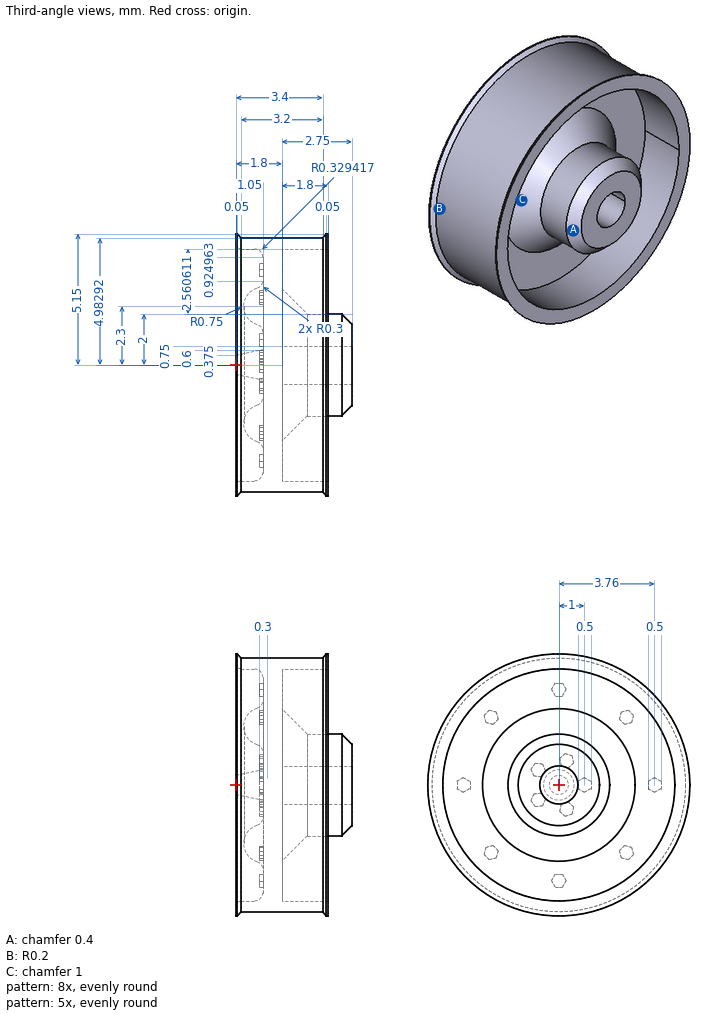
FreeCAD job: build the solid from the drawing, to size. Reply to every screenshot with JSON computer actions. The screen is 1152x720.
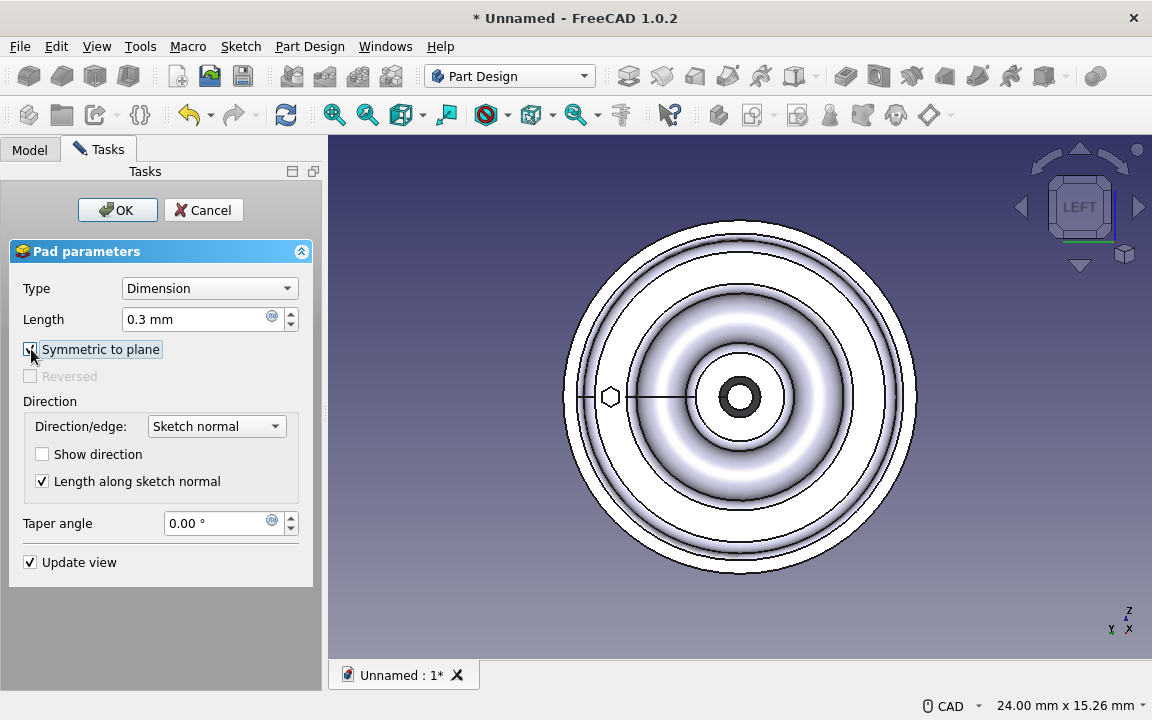
{"action": "left_click", "coordinate": [118, 210]}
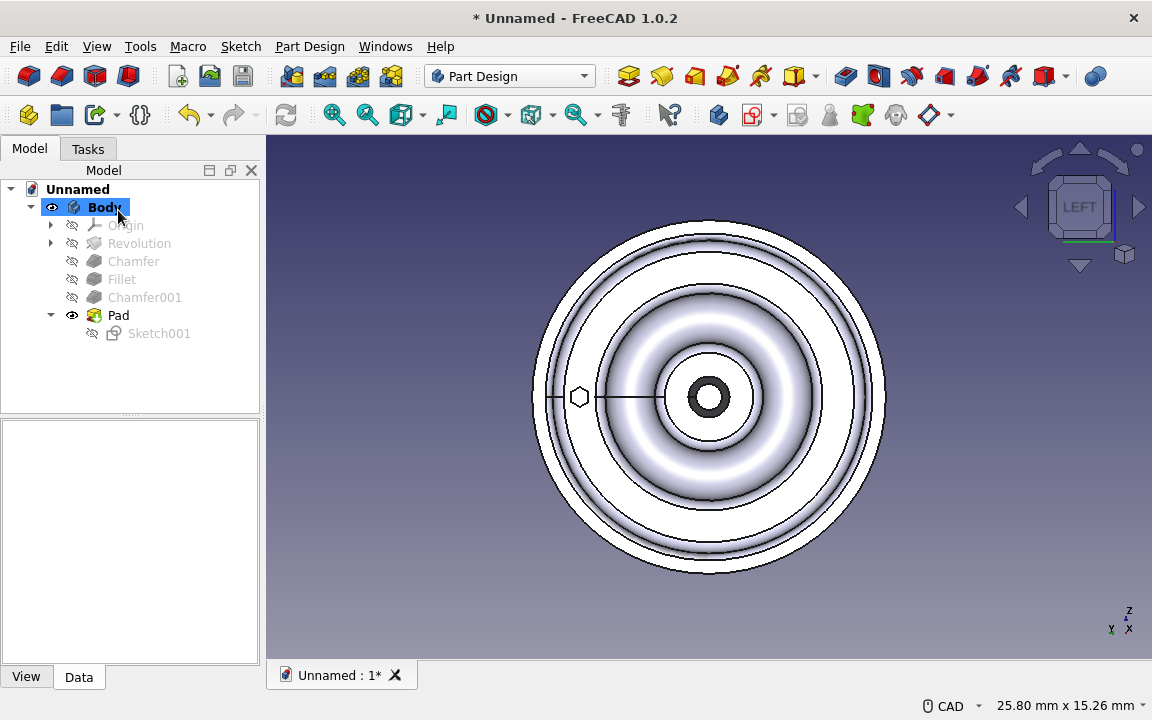
{"action": "left_click", "coordinate": [117, 315]}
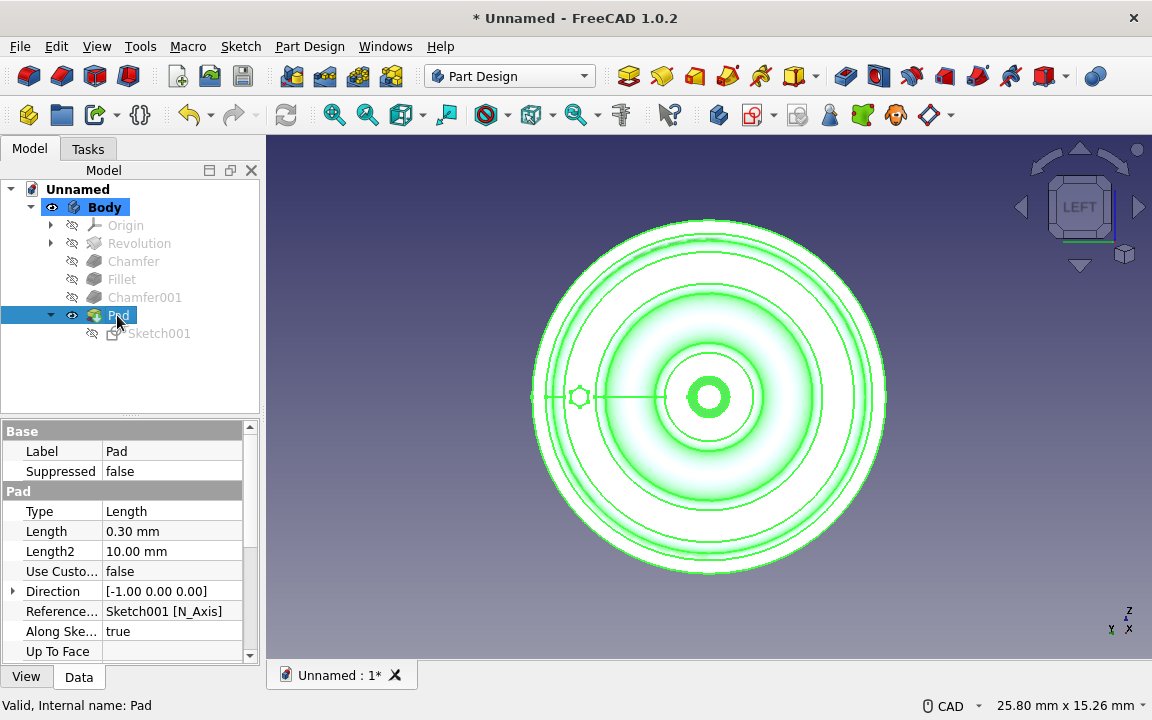
{"action": "left_click", "coordinate": [358, 76]}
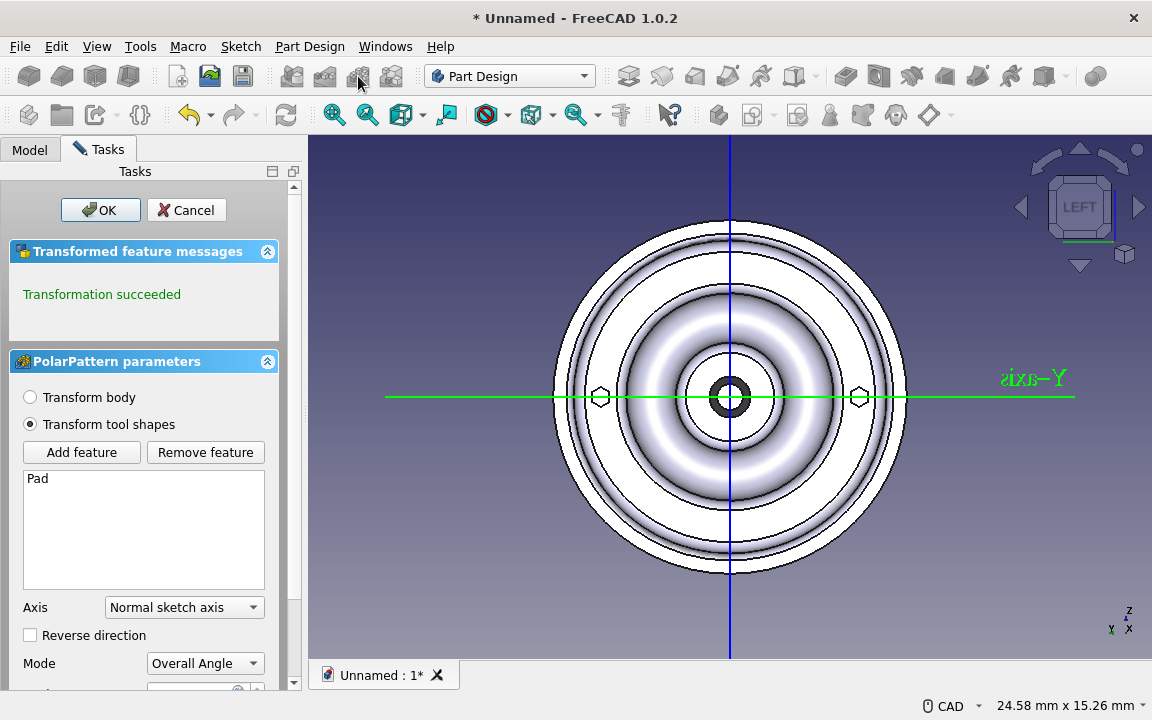
{"action": "left_click", "coordinate": [185, 608]}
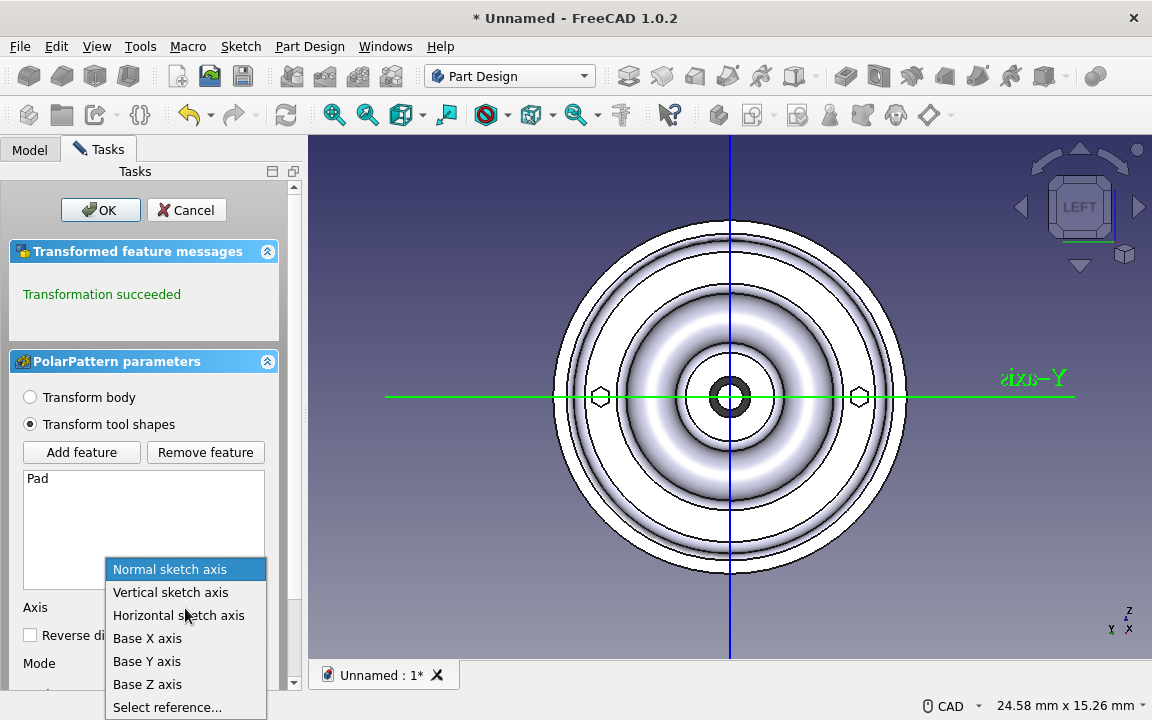
{"action": "left_click", "coordinate": [184, 638]}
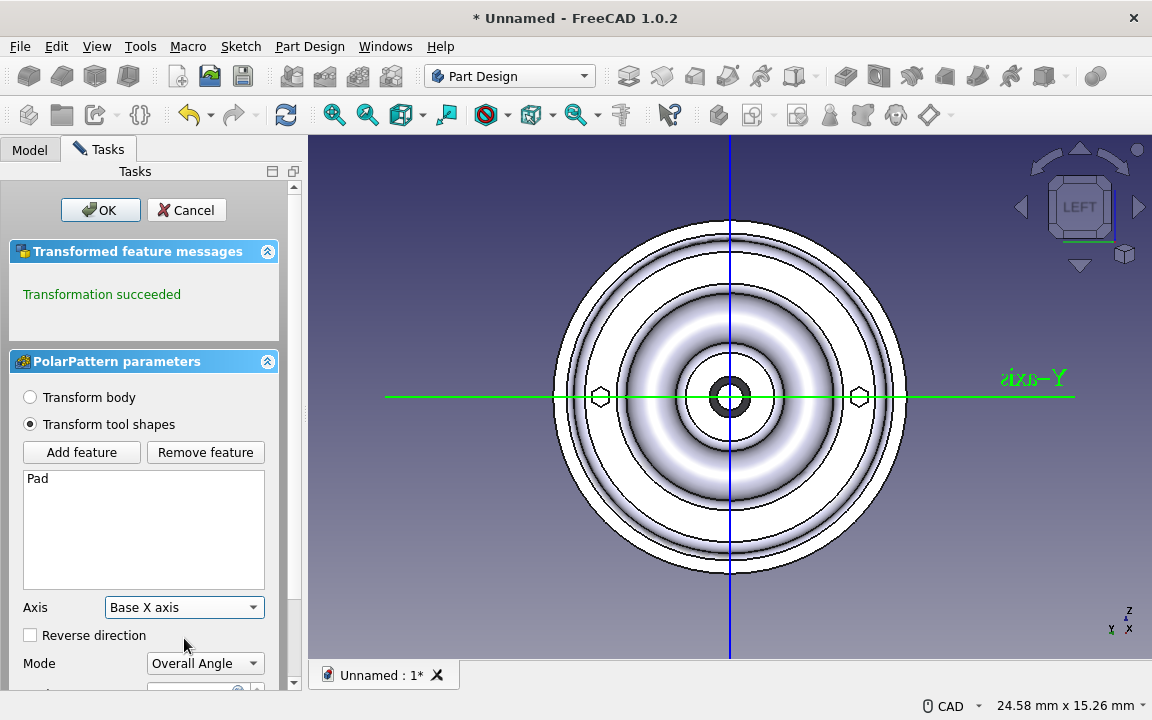
{"action": "scroll", "coordinate": [294, 436], "scroll_direction": "down", "scroll_amount": 2}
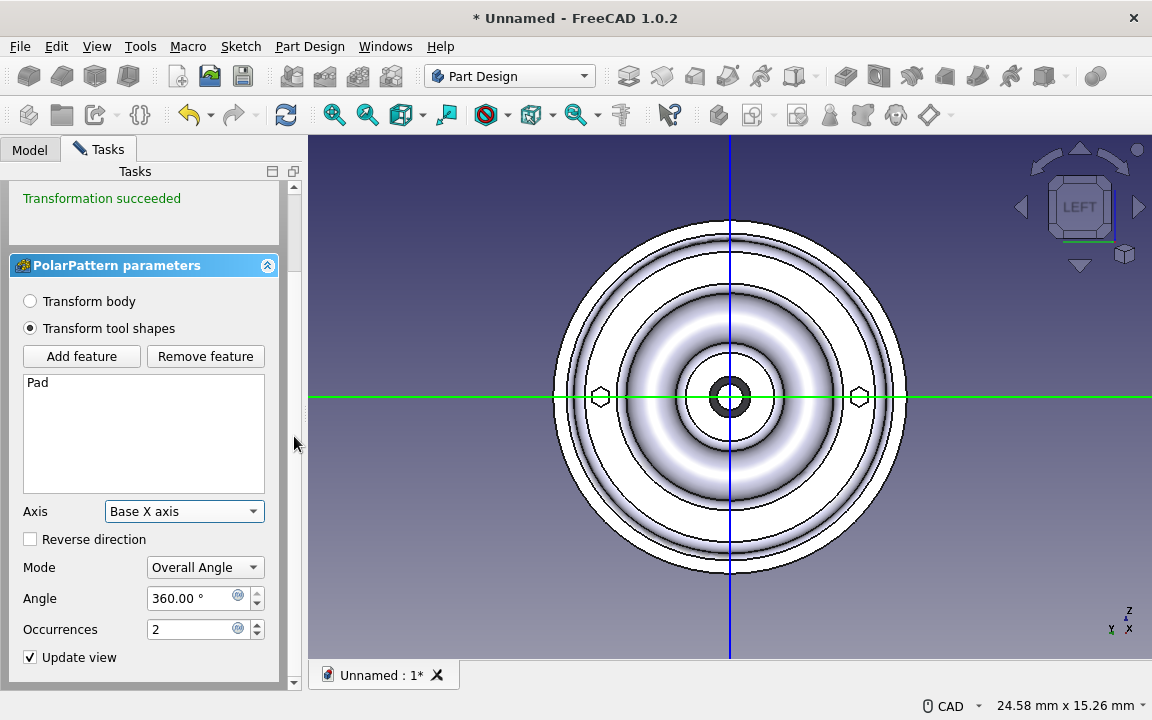
{"action": "triple_click", "coordinate": [199, 630]}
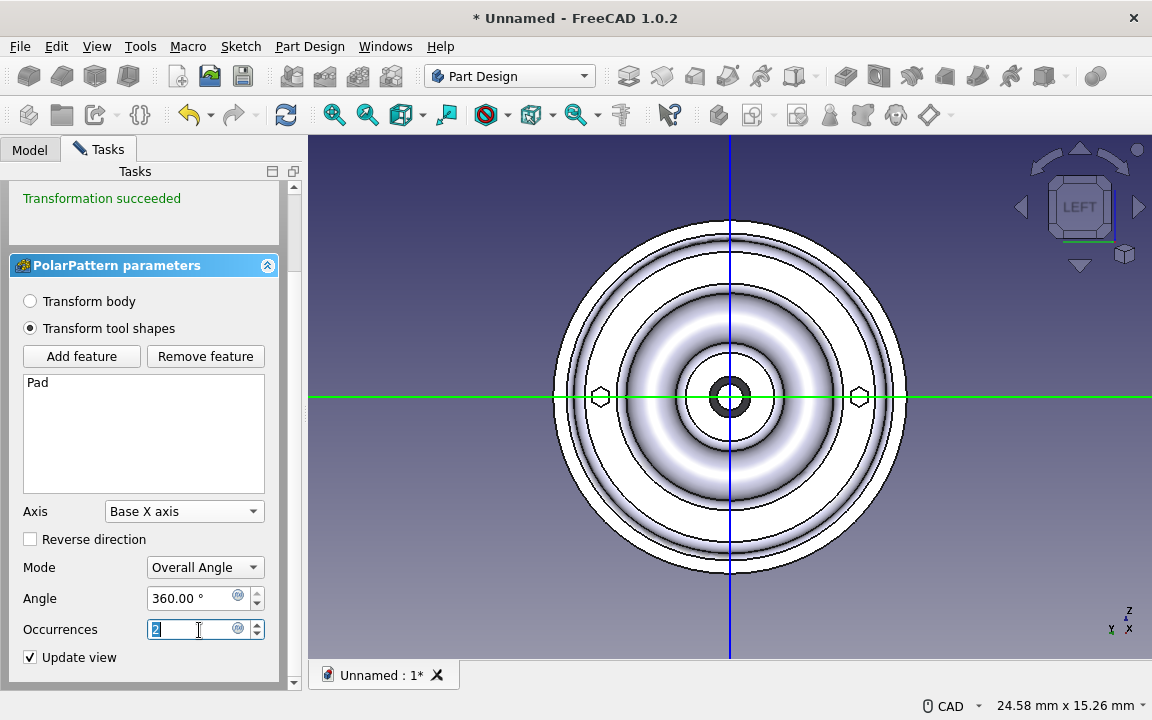
{"action": "type", "text": "8"}
{"action": "key", "text": "Tab"}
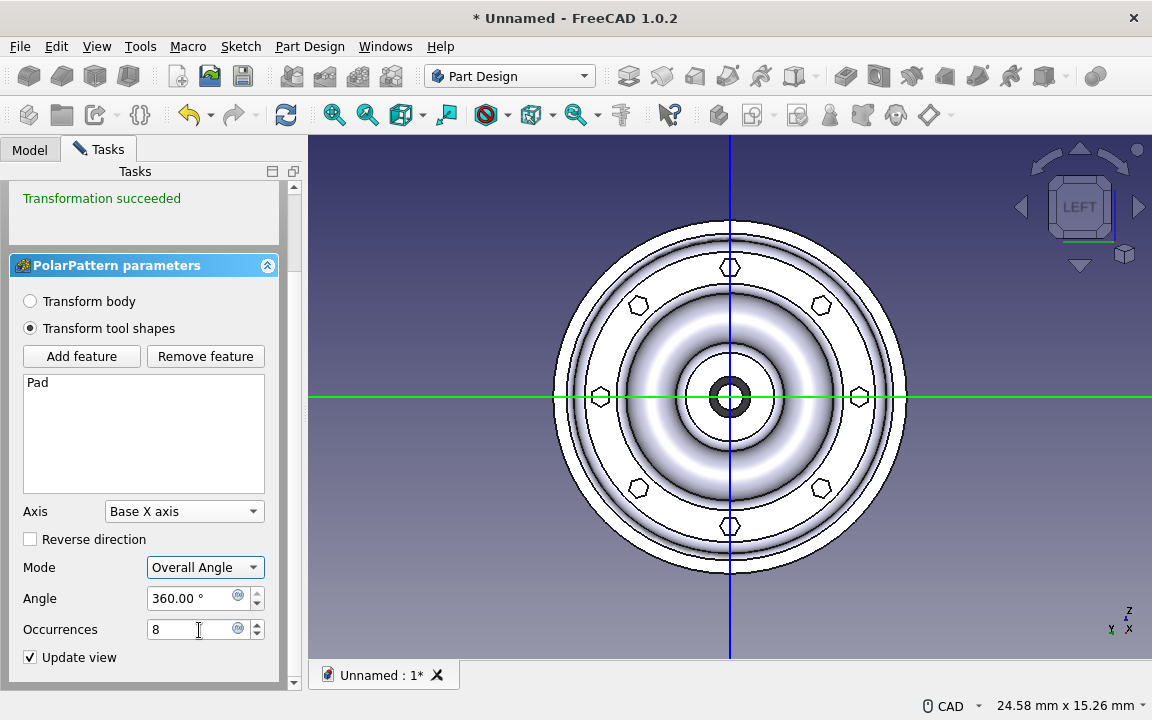
{"action": "scroll", "coordinate": [294, 436], "scroll_direction": "up", "scroll_amount": 3}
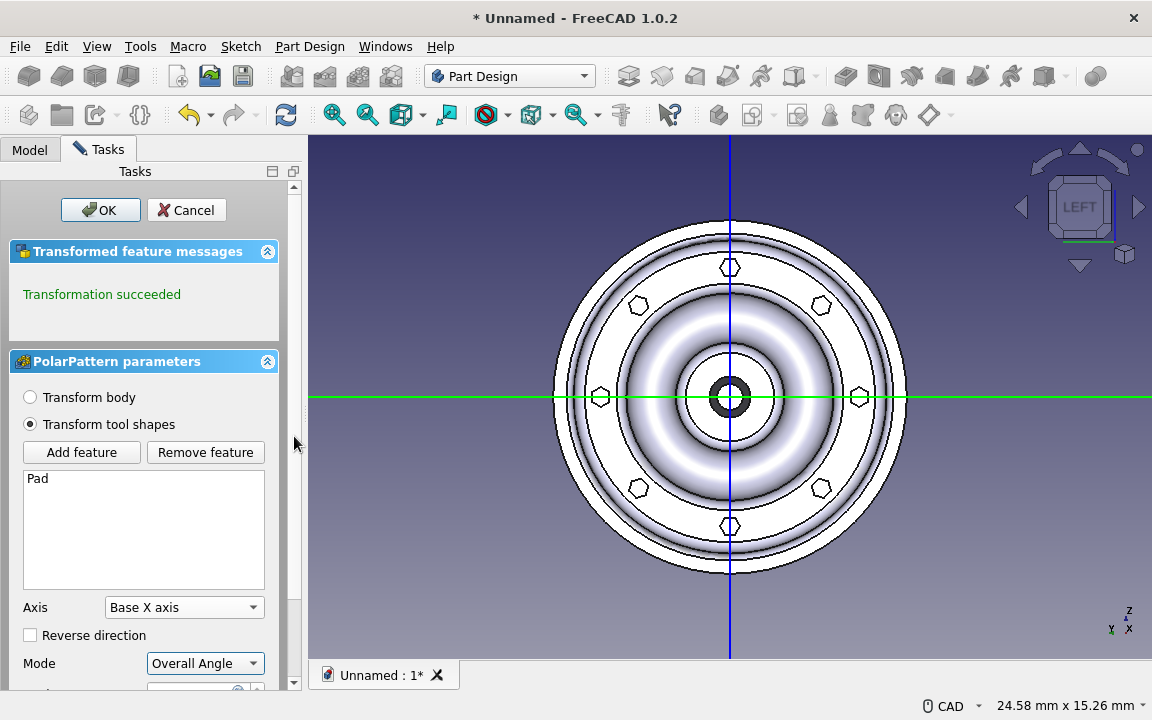
{"action": "left_click", "coordinate": [101, 210]}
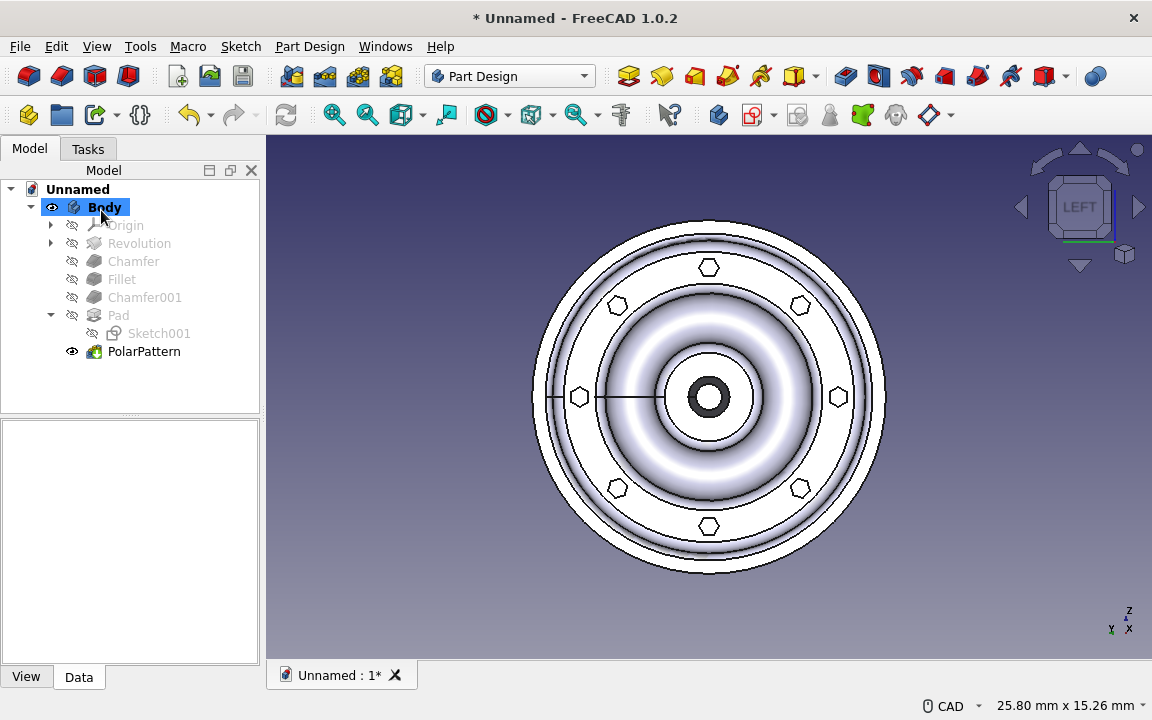
{"action": "left_click", "coordinate": [751, 271]}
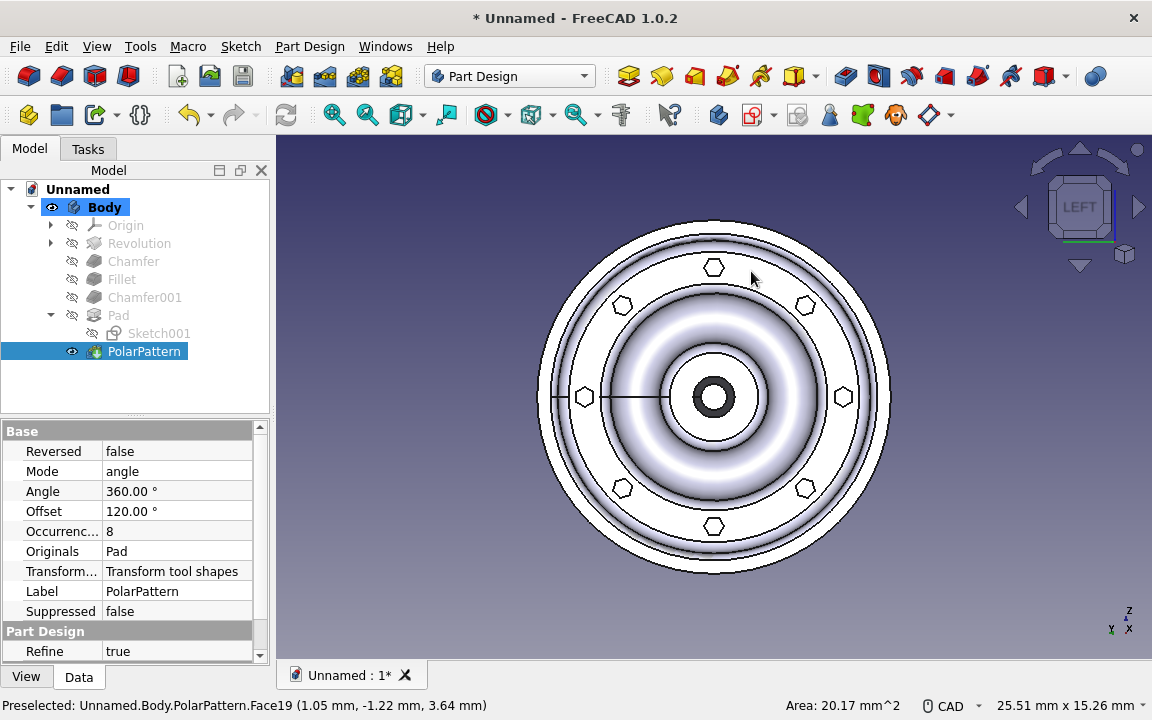
{"action": "left_click", "coordinate": [752, 116]}